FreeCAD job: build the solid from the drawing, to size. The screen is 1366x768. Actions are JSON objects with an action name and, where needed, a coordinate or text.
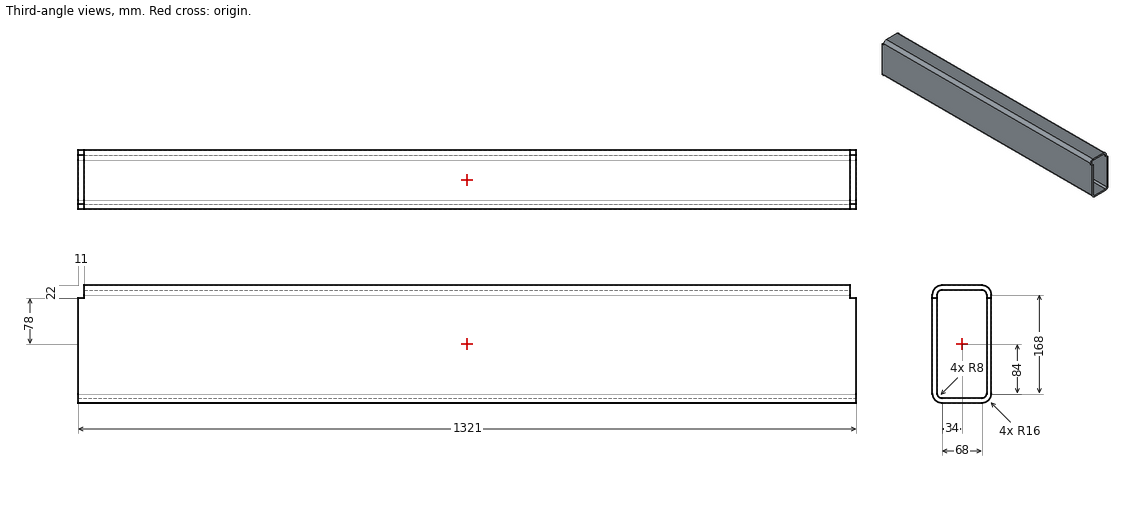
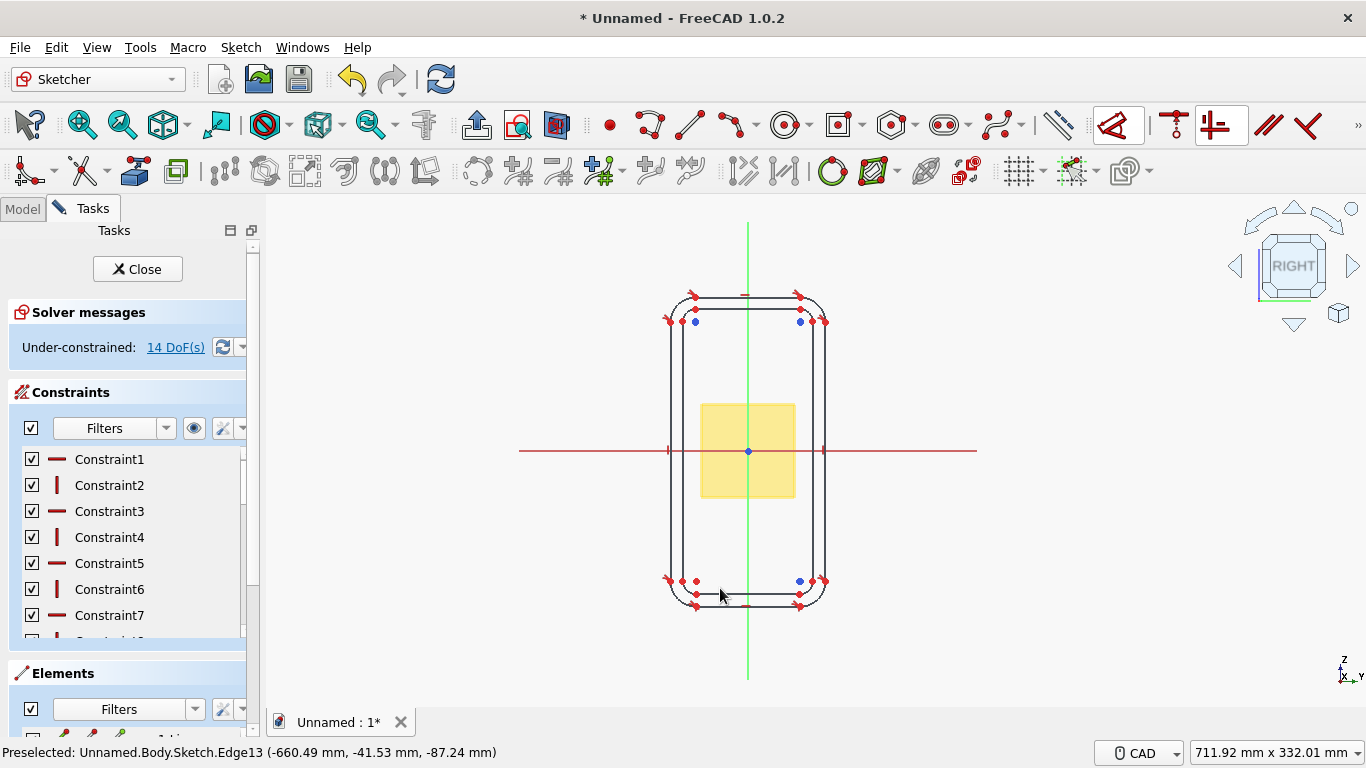
{"action": "left_click", "coordinate": [684, 300]}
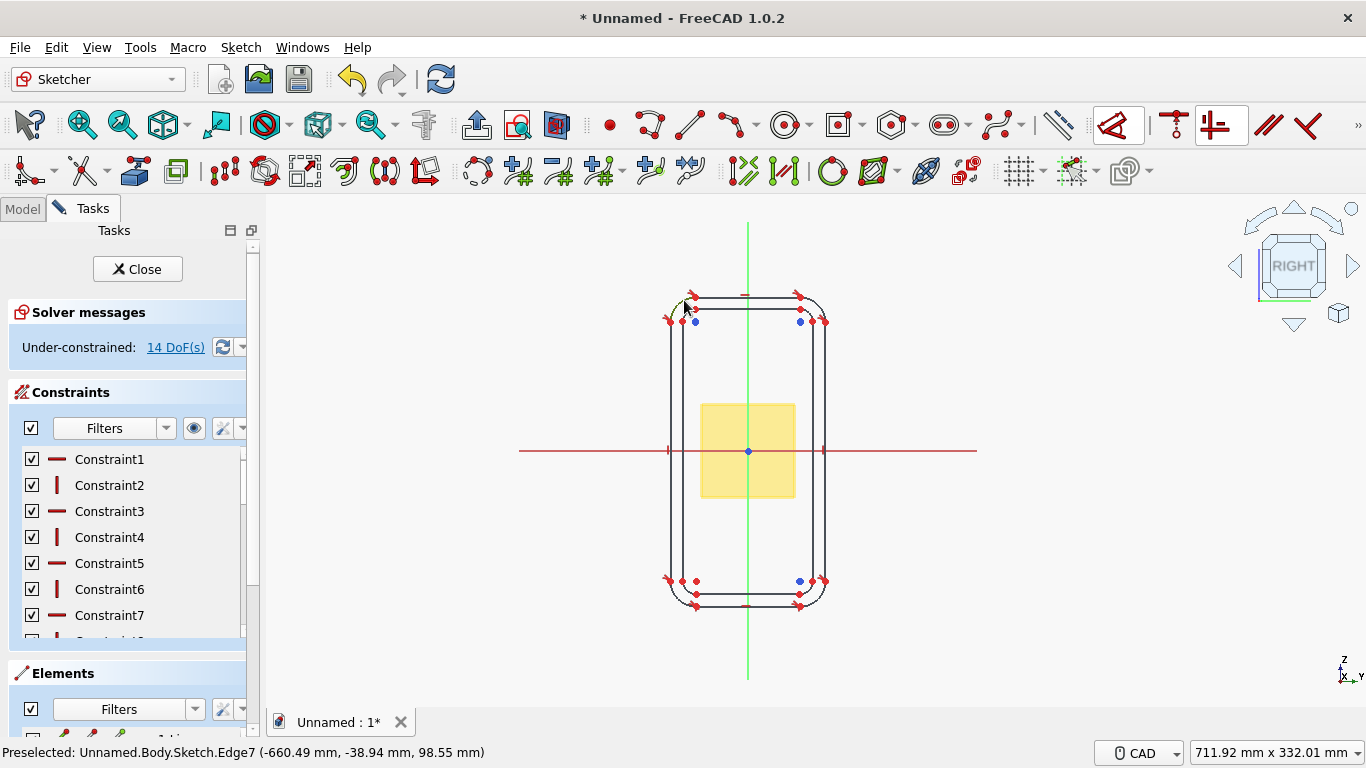
{"action": "scroll", "coordinate": [687, 313], "scroll_direction": "up", "scroll_amount": 2}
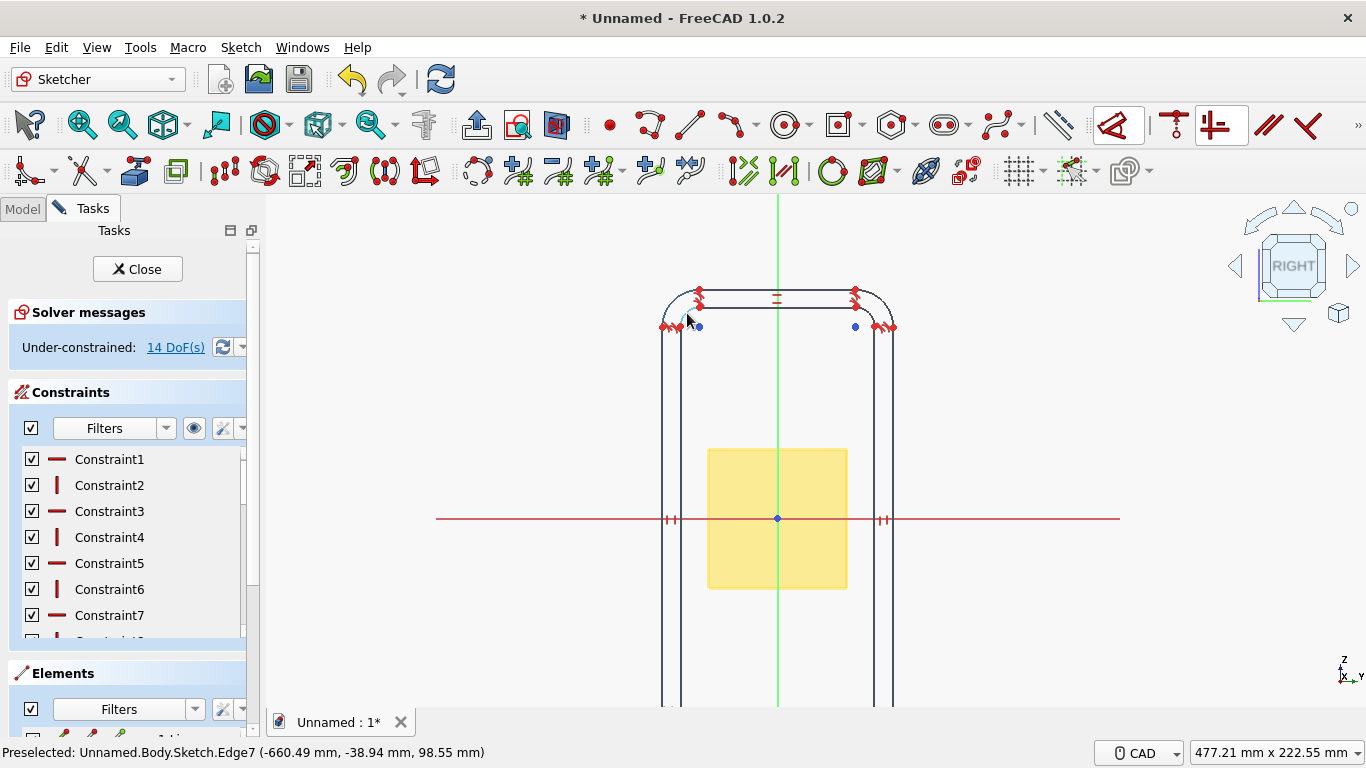
{"action": "left_click", "coordinate": [686, 313]}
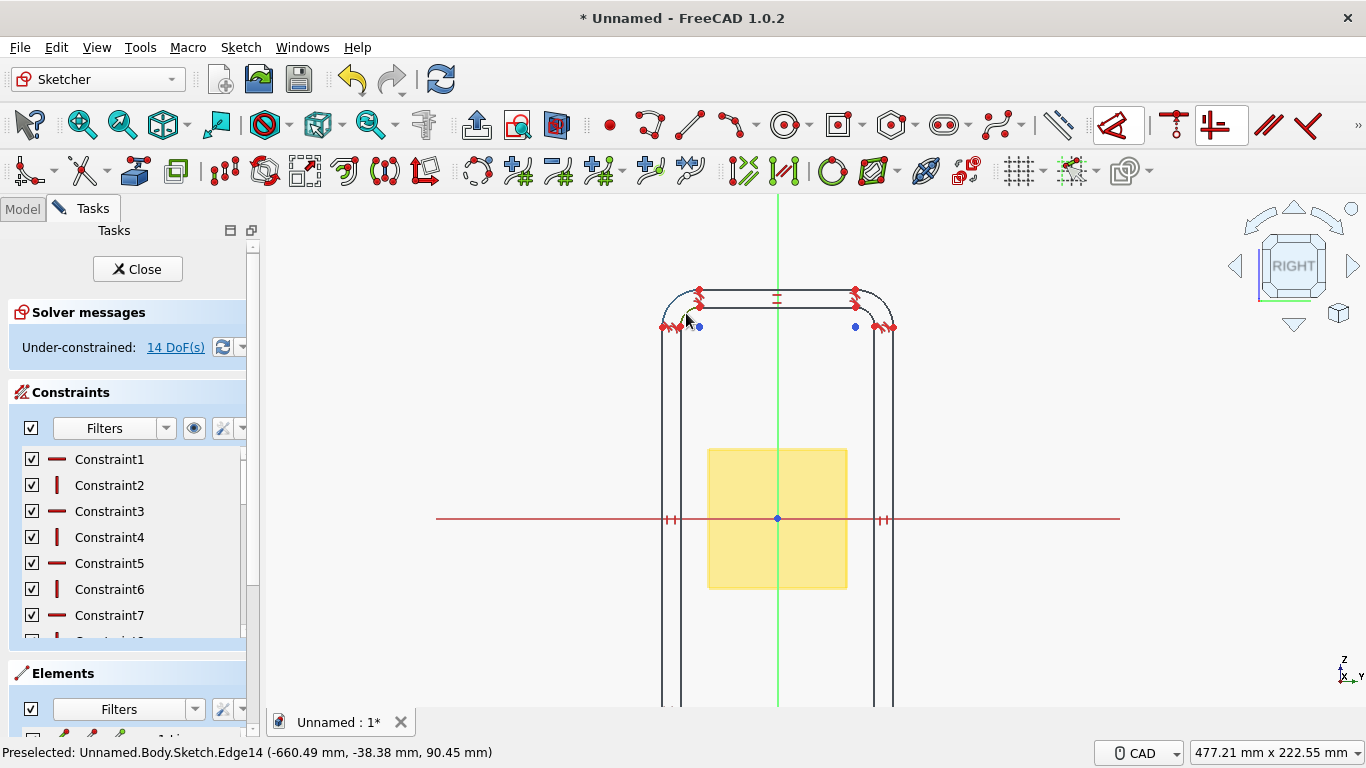
{"action": "key", "text": "c"}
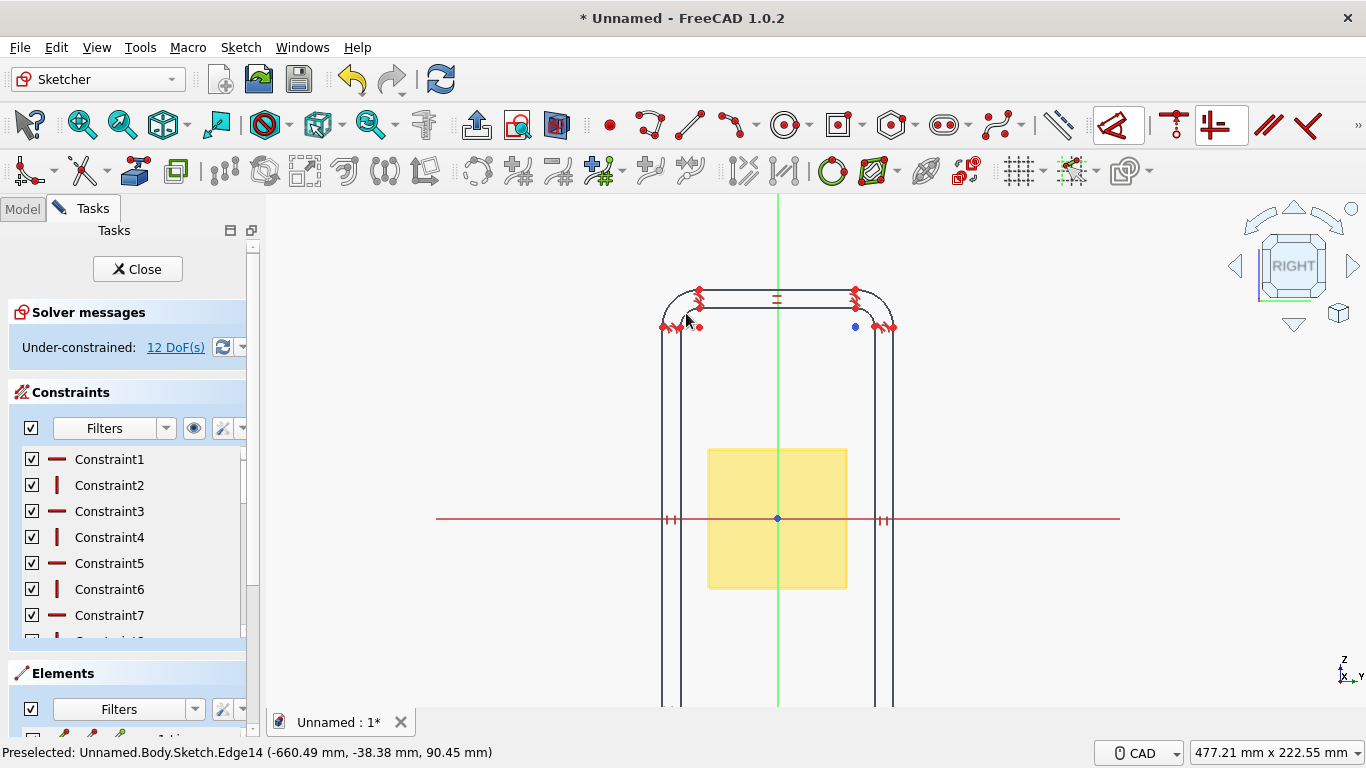
{"action": "left_click", "coordinate": [889, 310]}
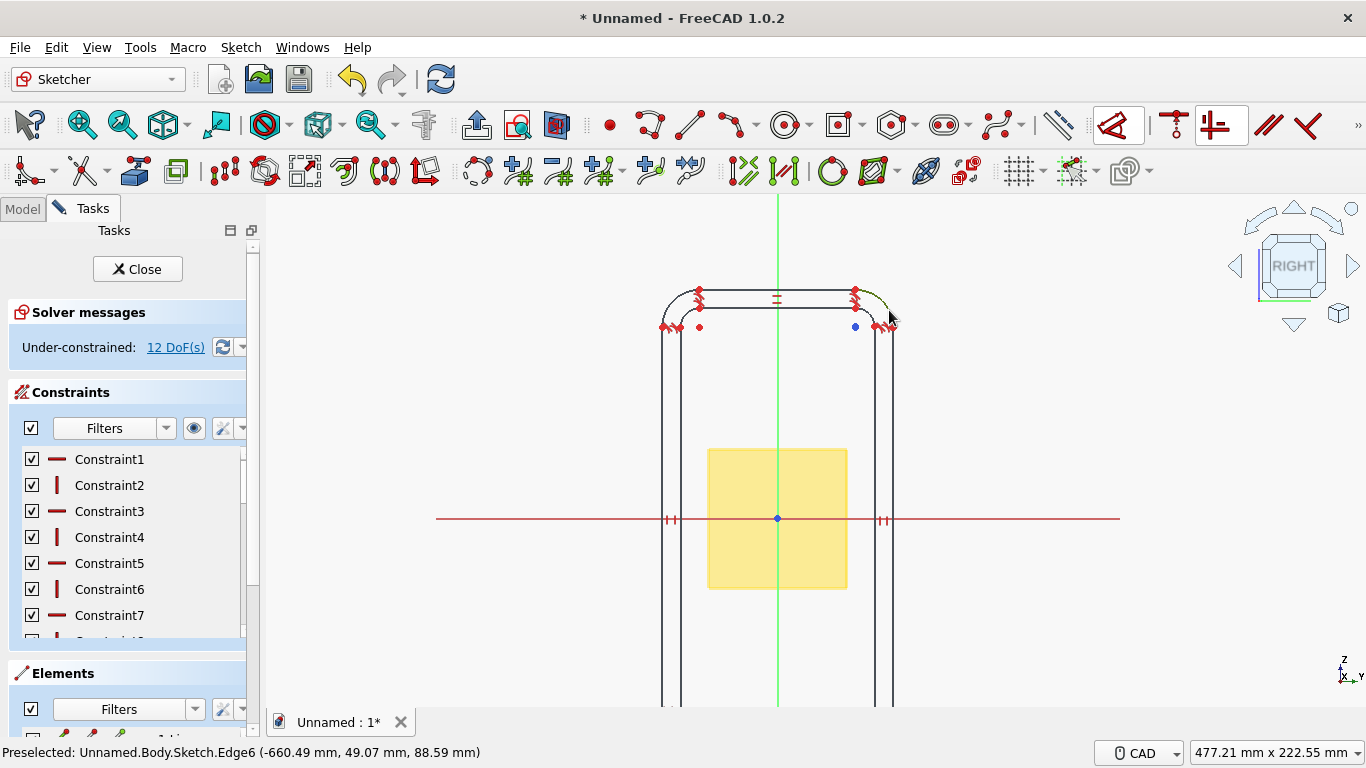
{"action": "left_click", "coordinate": [869, 314]}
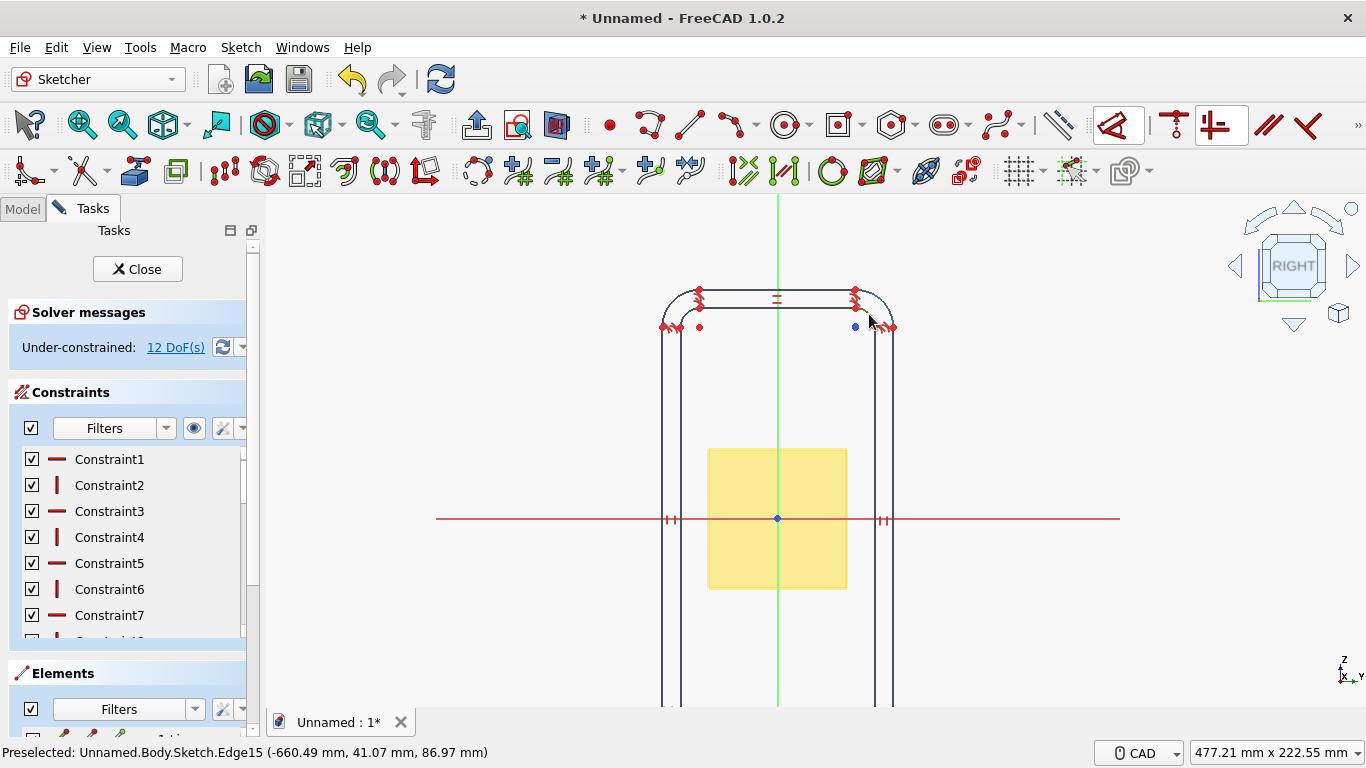
{"action": "key", "text": "c"}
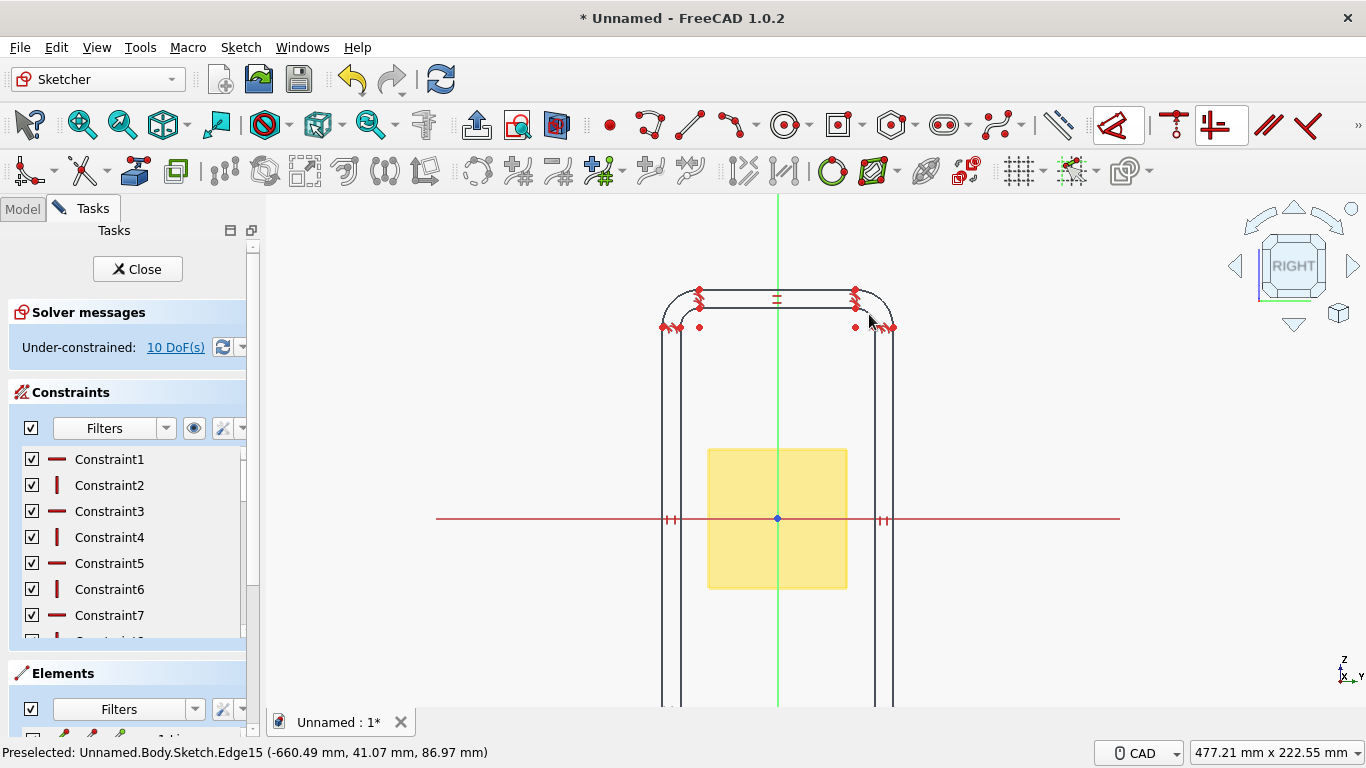
{"action": "scroll", "coordinate": [686, 311], "scroll_direction": "down", "scroll_amount": 2}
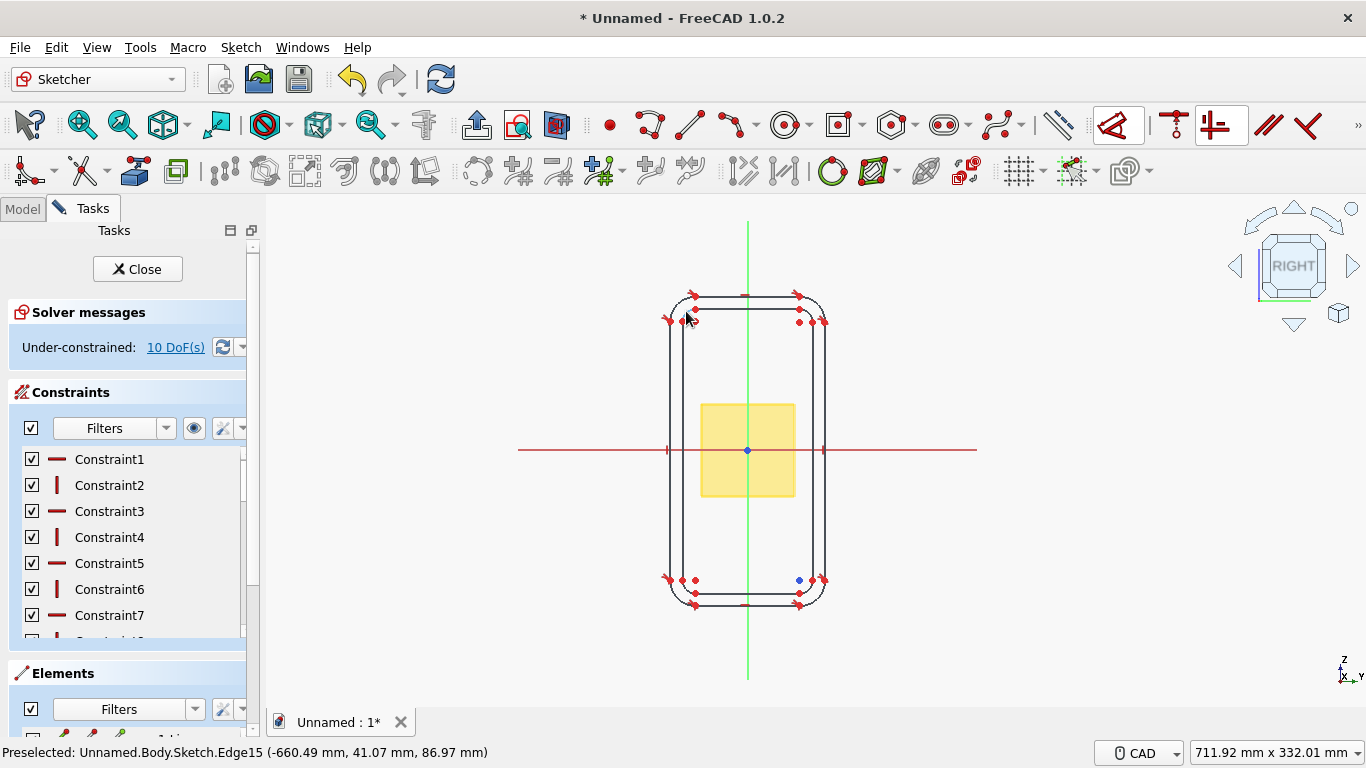
{"action": "left_click", "coordinate": [811, 603]}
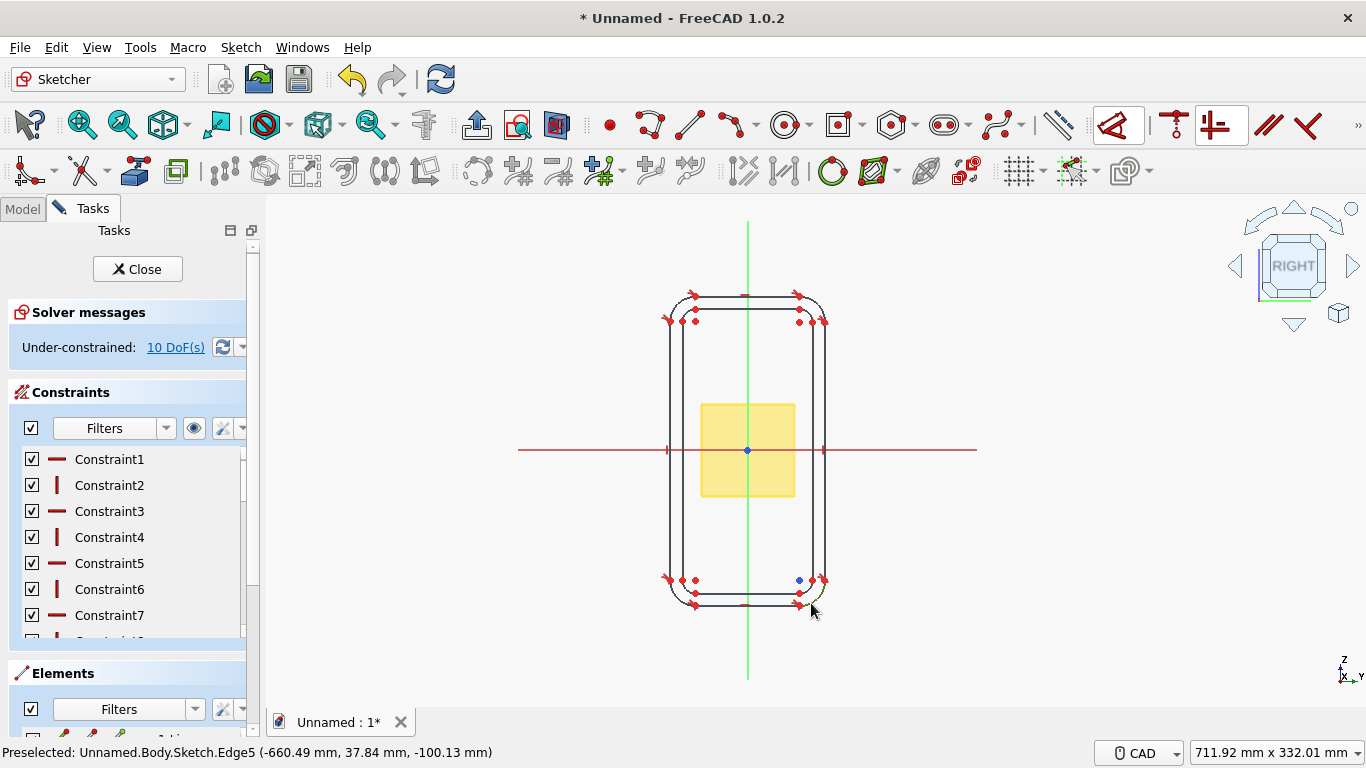
{"action": "left_click", "coordinate": [822, 311]}